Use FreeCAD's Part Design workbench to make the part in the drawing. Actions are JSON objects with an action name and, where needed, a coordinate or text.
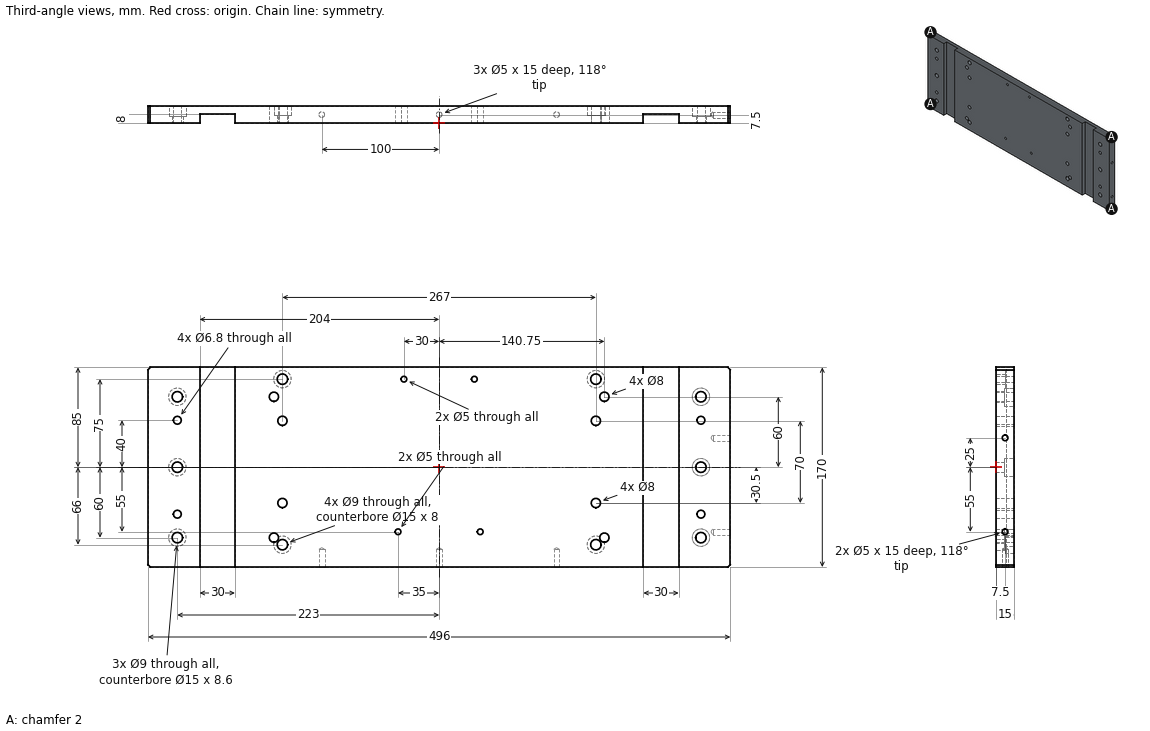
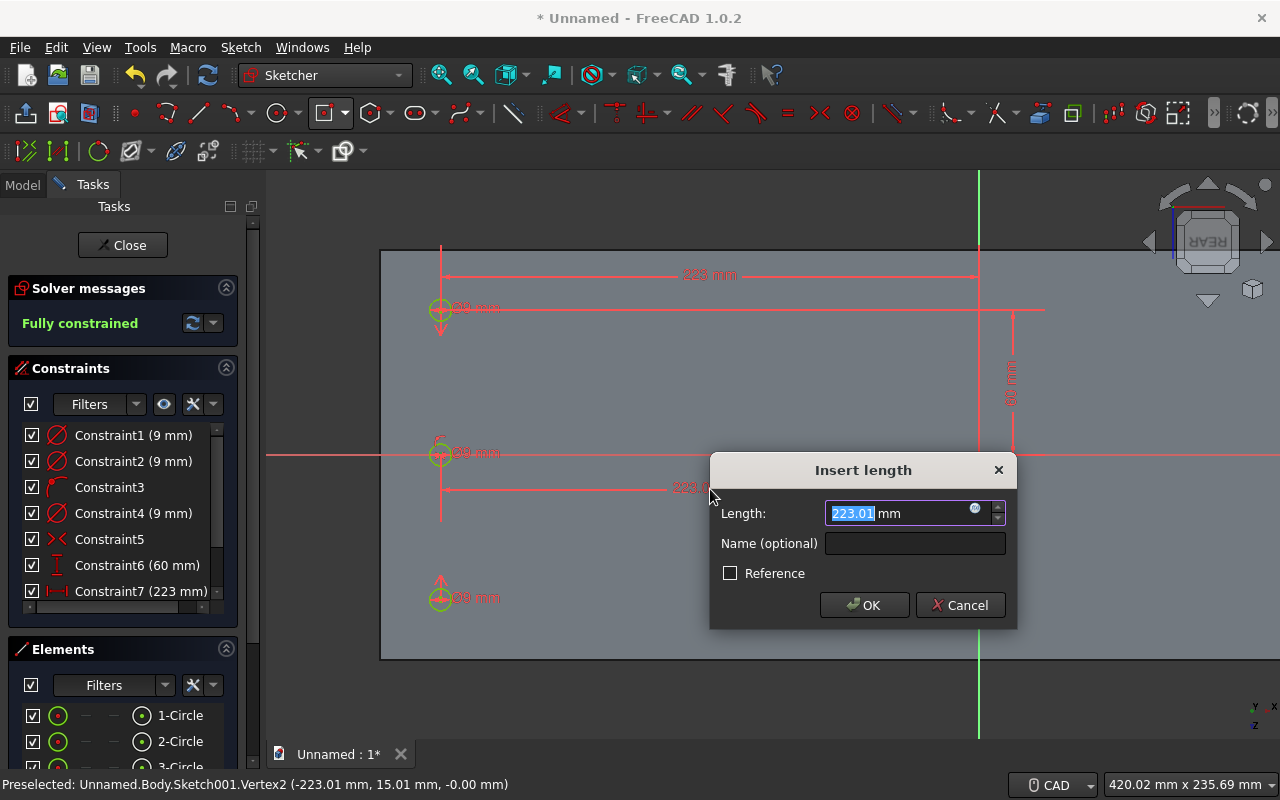
{"action": "type", "text": "223"}
{"action": "key", "text": "Return"}
{"action": "key", "text": "Escape"}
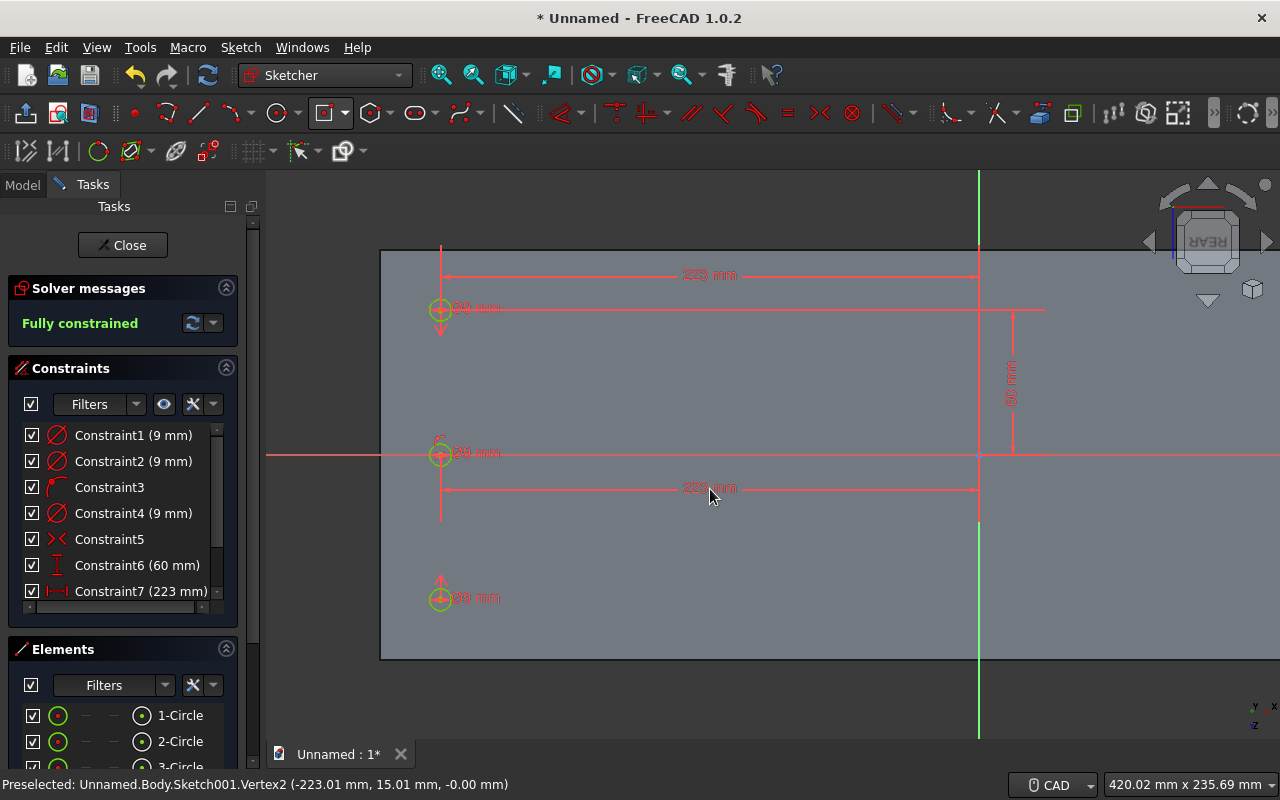
{"action": "left_click", "coordinate": [123, 245]}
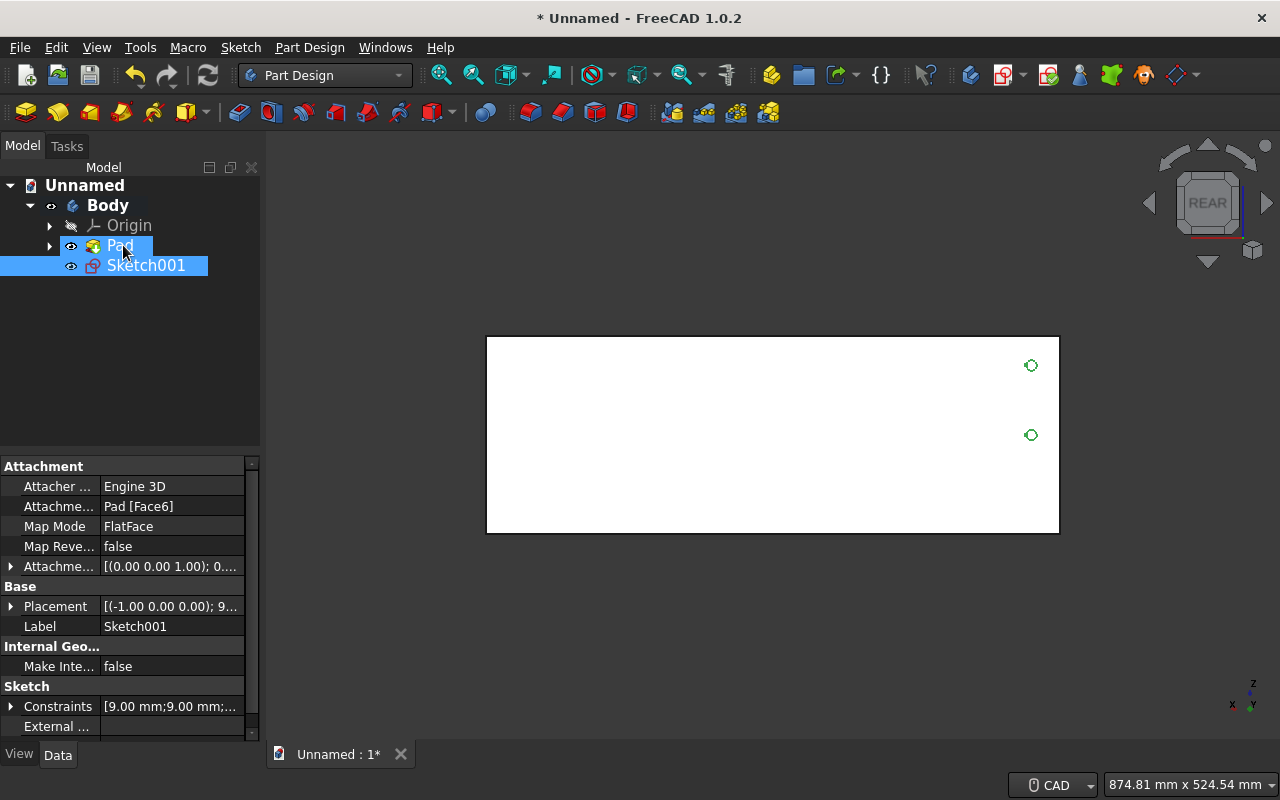
{"action": "left_click", "coordinate": [272, 112]}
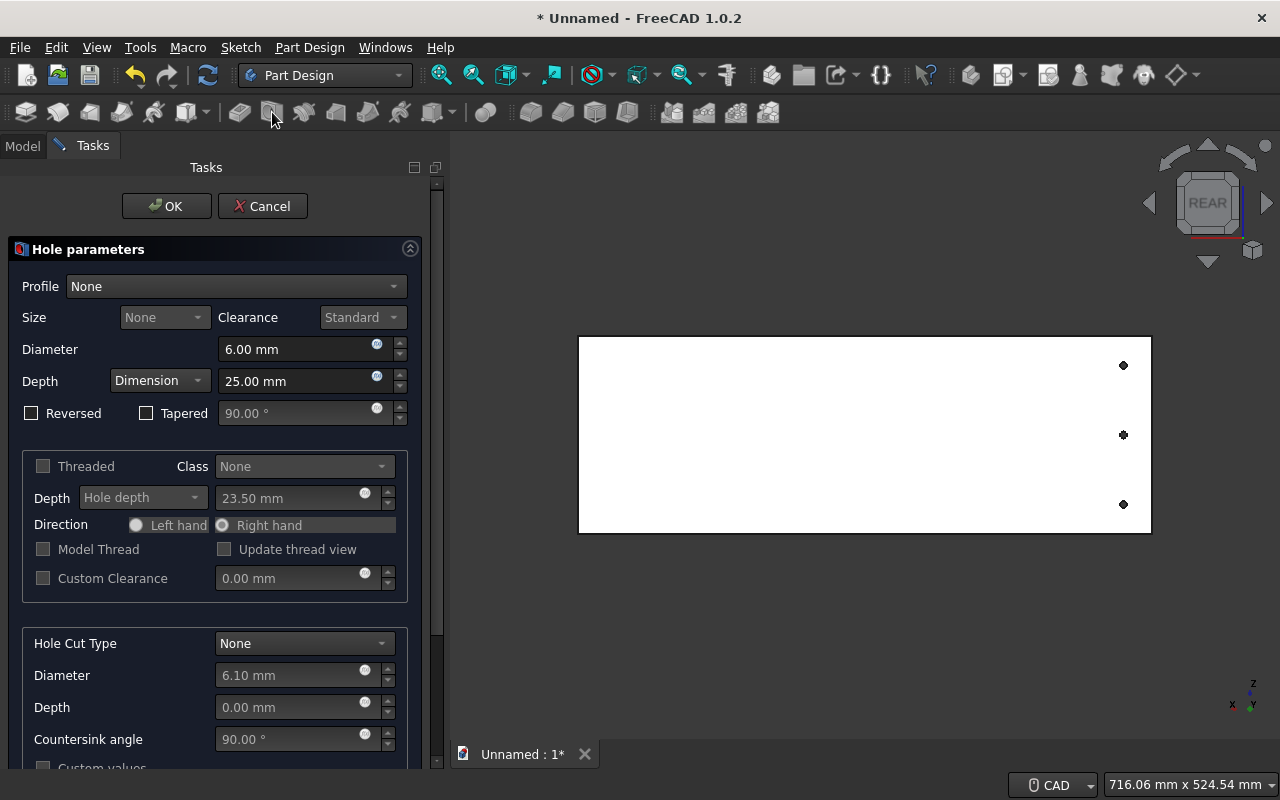
{"action": "triple_click", "coordinate": [305, 349]}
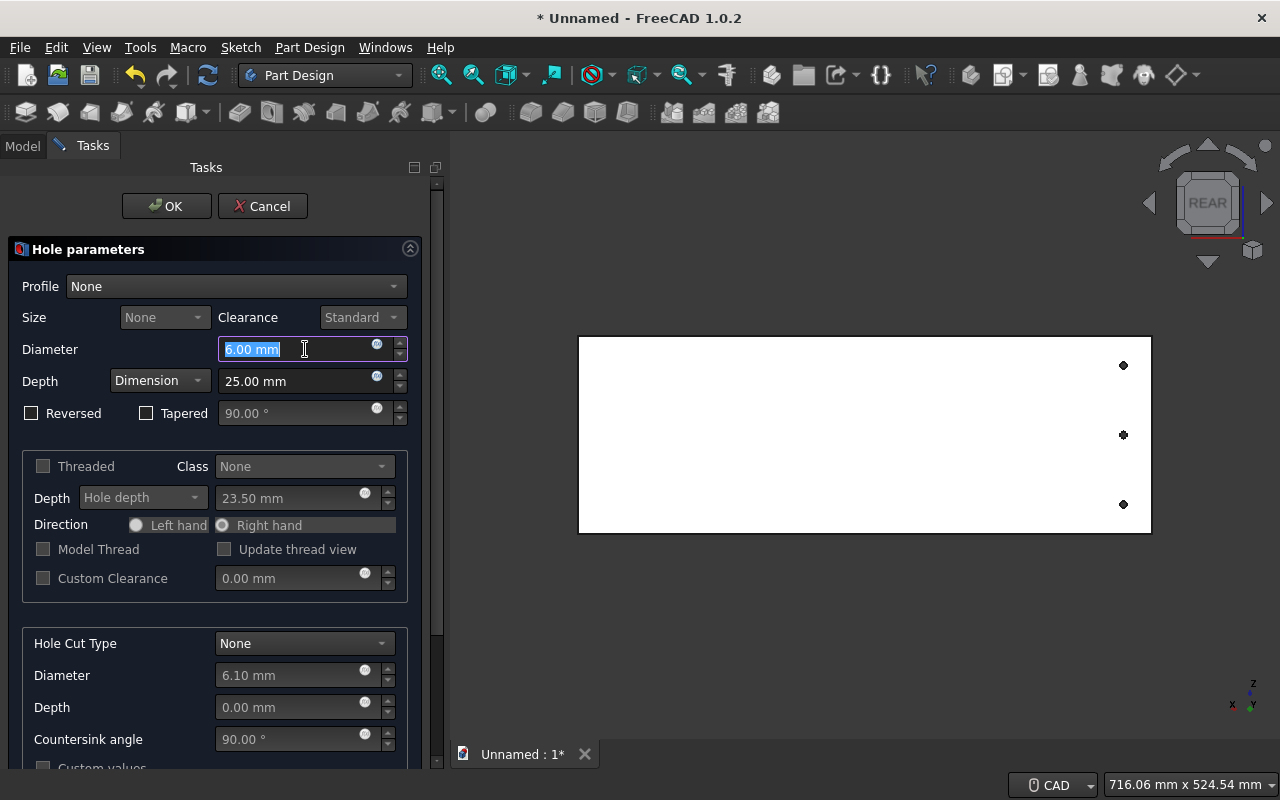
{"action": "type", "text": "9"}
{"action": "key", "text": "Tab"}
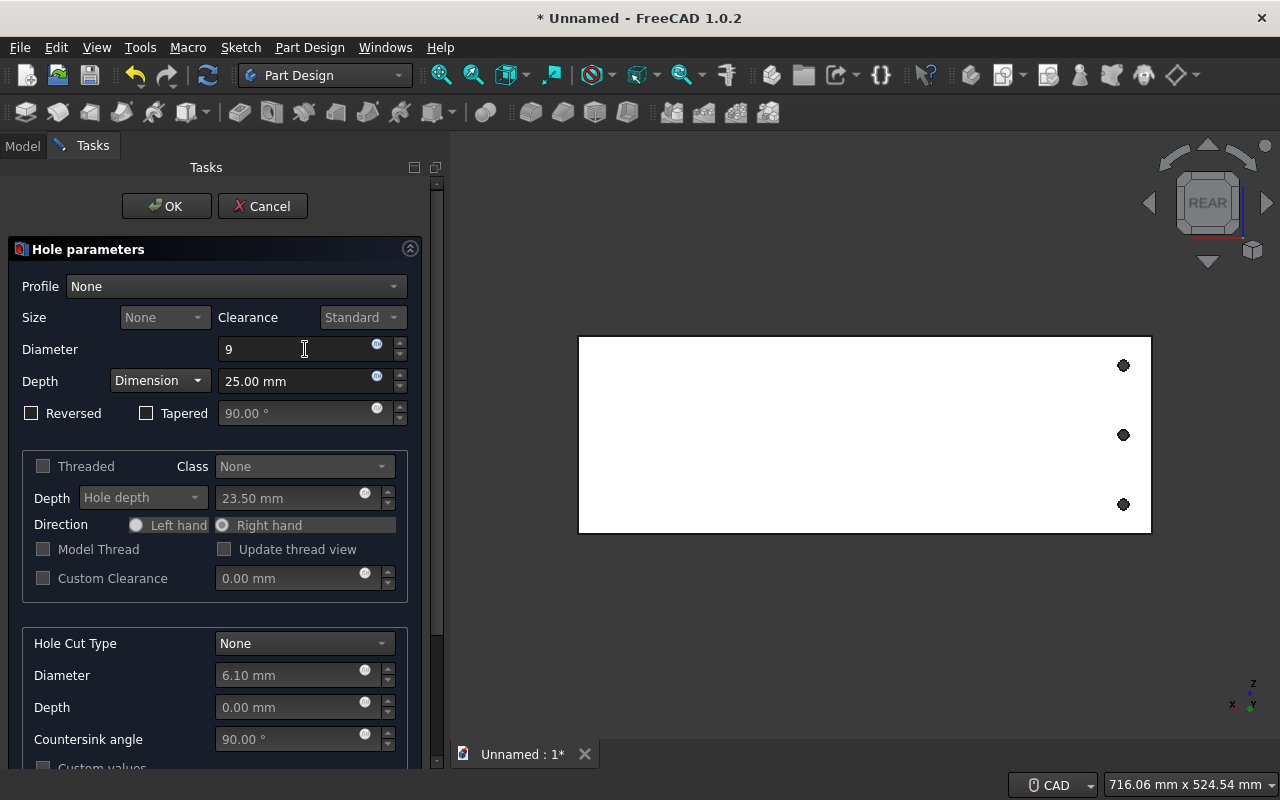
{"action": "left_click", "coordinate": [161, 380]}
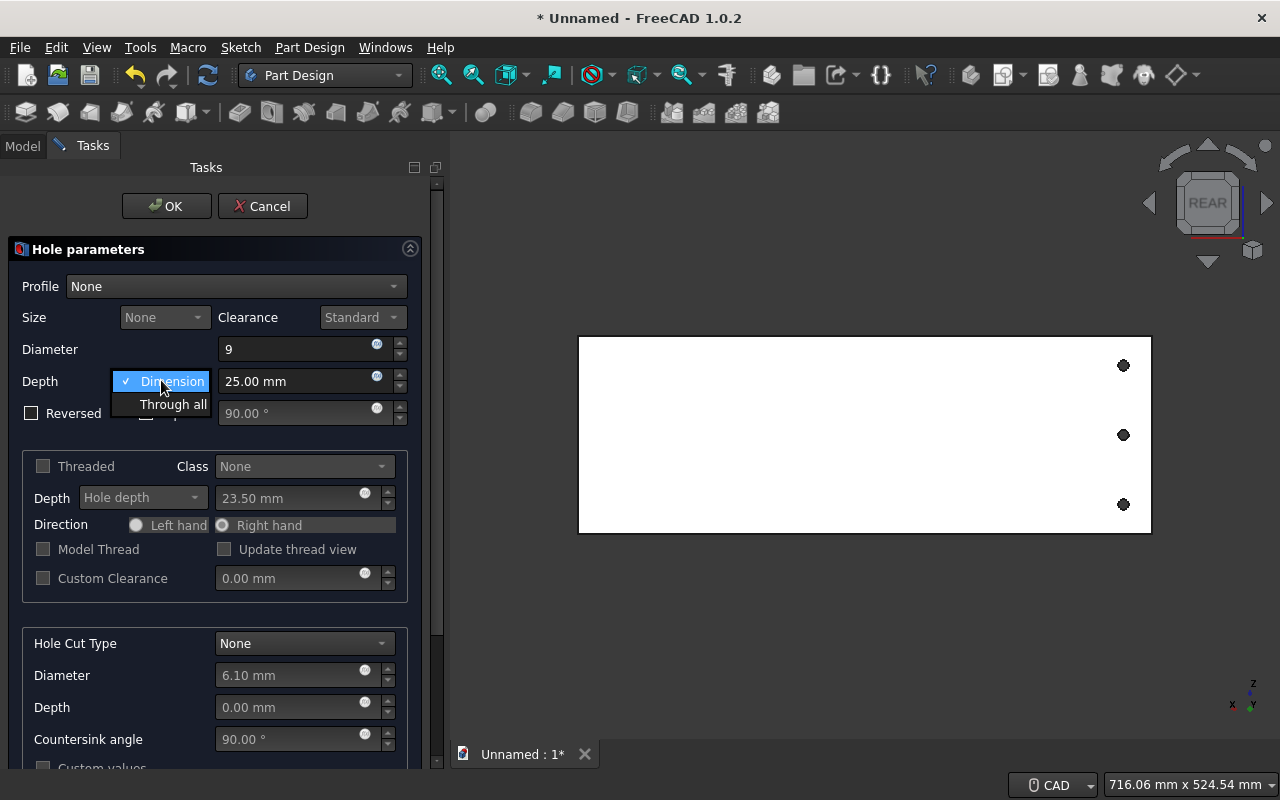
{"action": "left_click", "coordinate": [160, 404]}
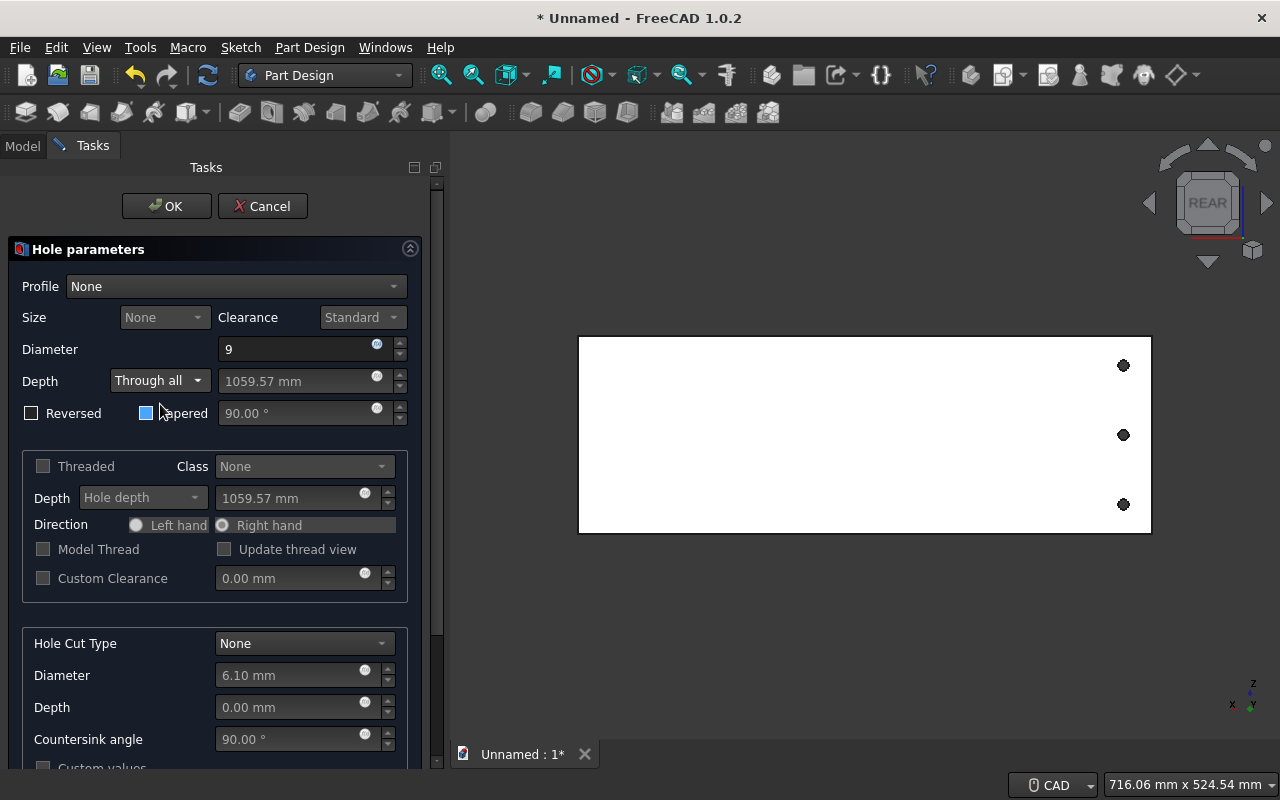
{"action": "left_click", "coordinate": [306, 644]}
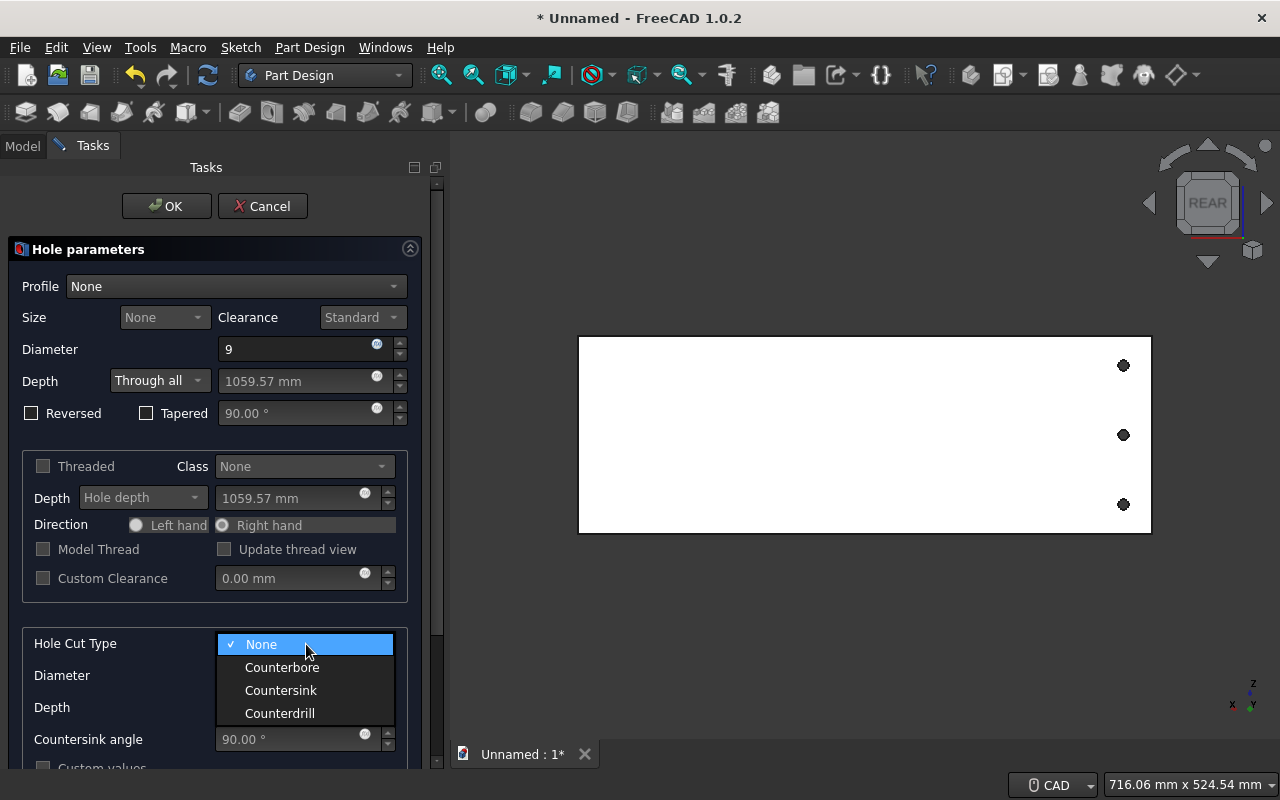
{"action": "left_click", "coordinate": [304, 668]}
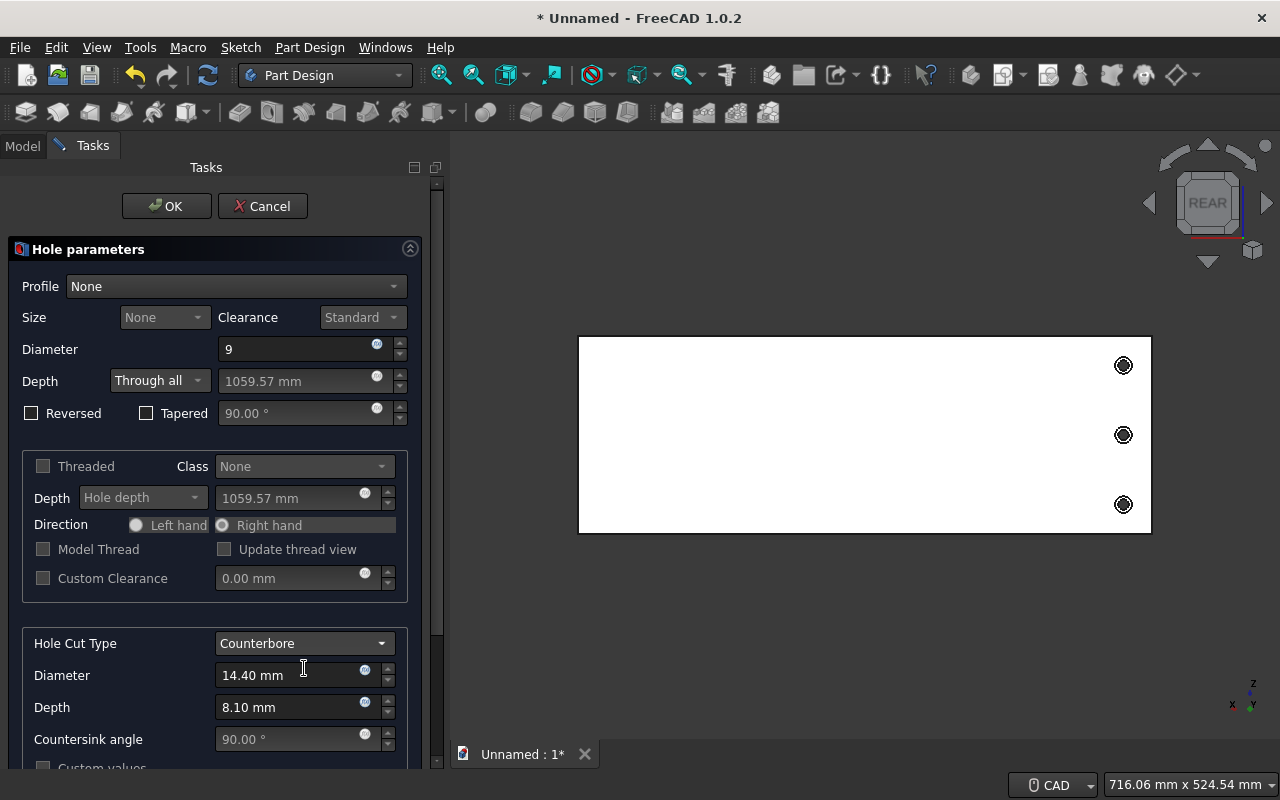
{"action": "triple_click", "coordinate": [298, 675]}